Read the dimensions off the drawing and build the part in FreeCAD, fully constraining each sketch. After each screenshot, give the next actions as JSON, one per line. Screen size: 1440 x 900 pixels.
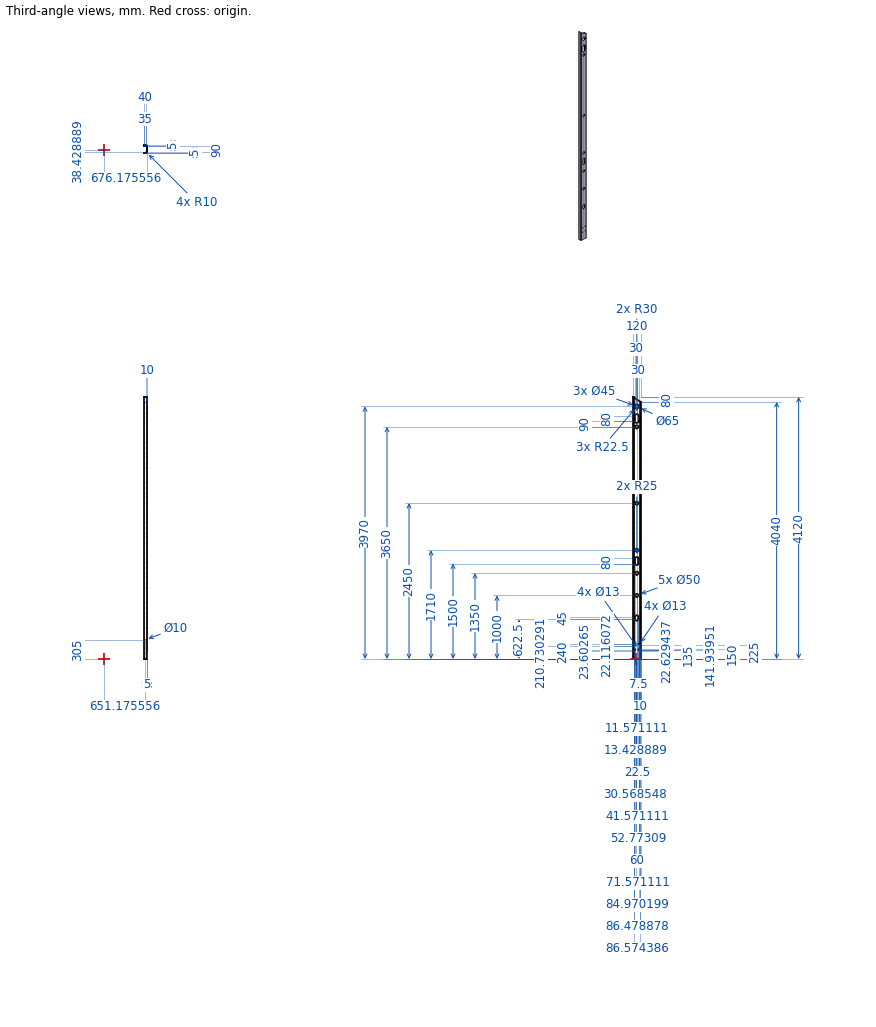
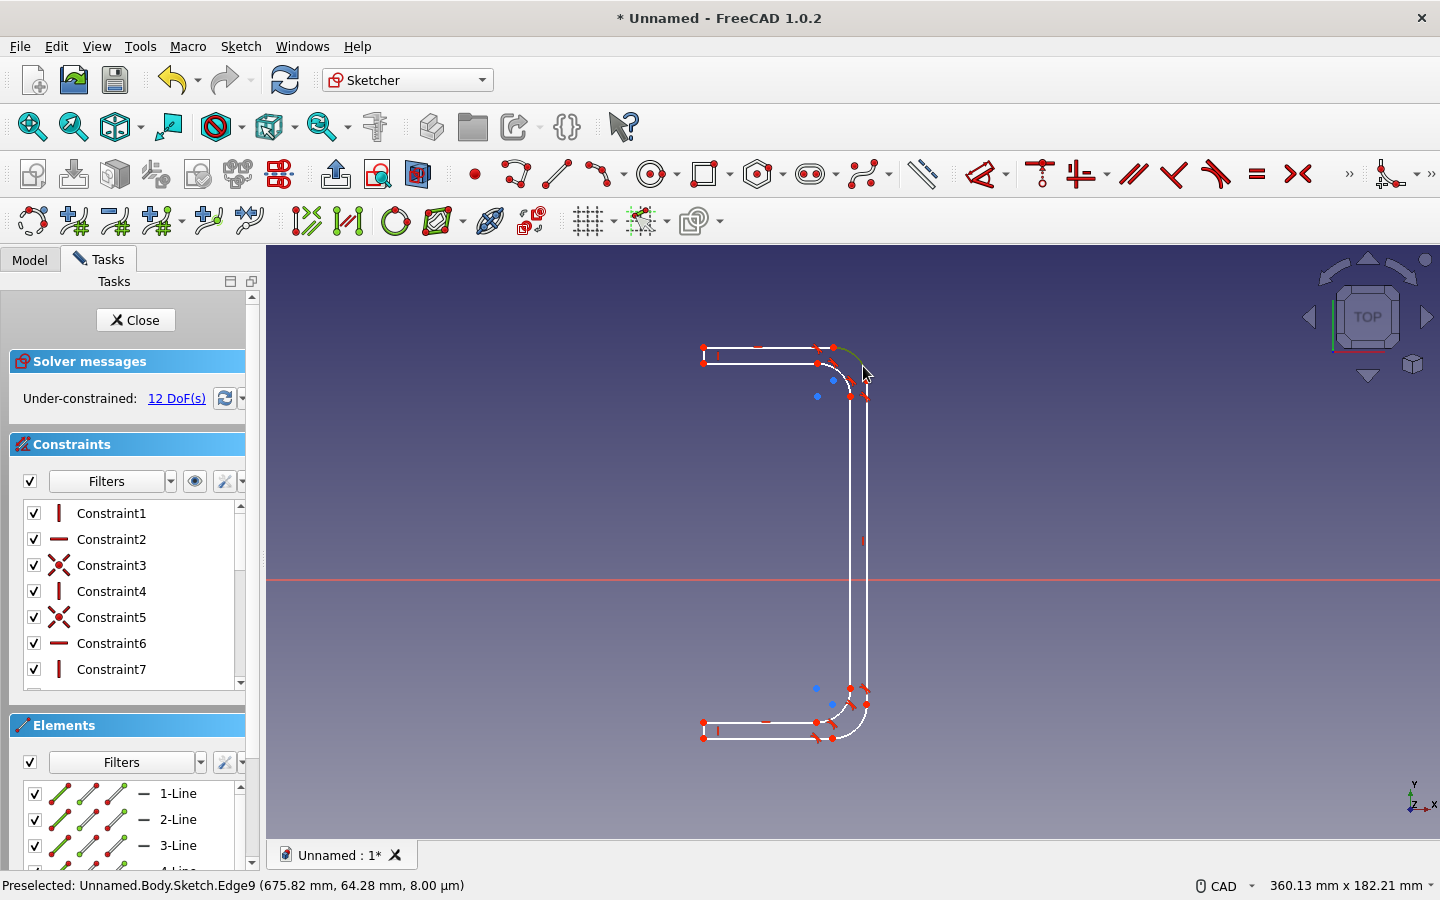
{"action": "left_click", "coordinate": [841, 373]}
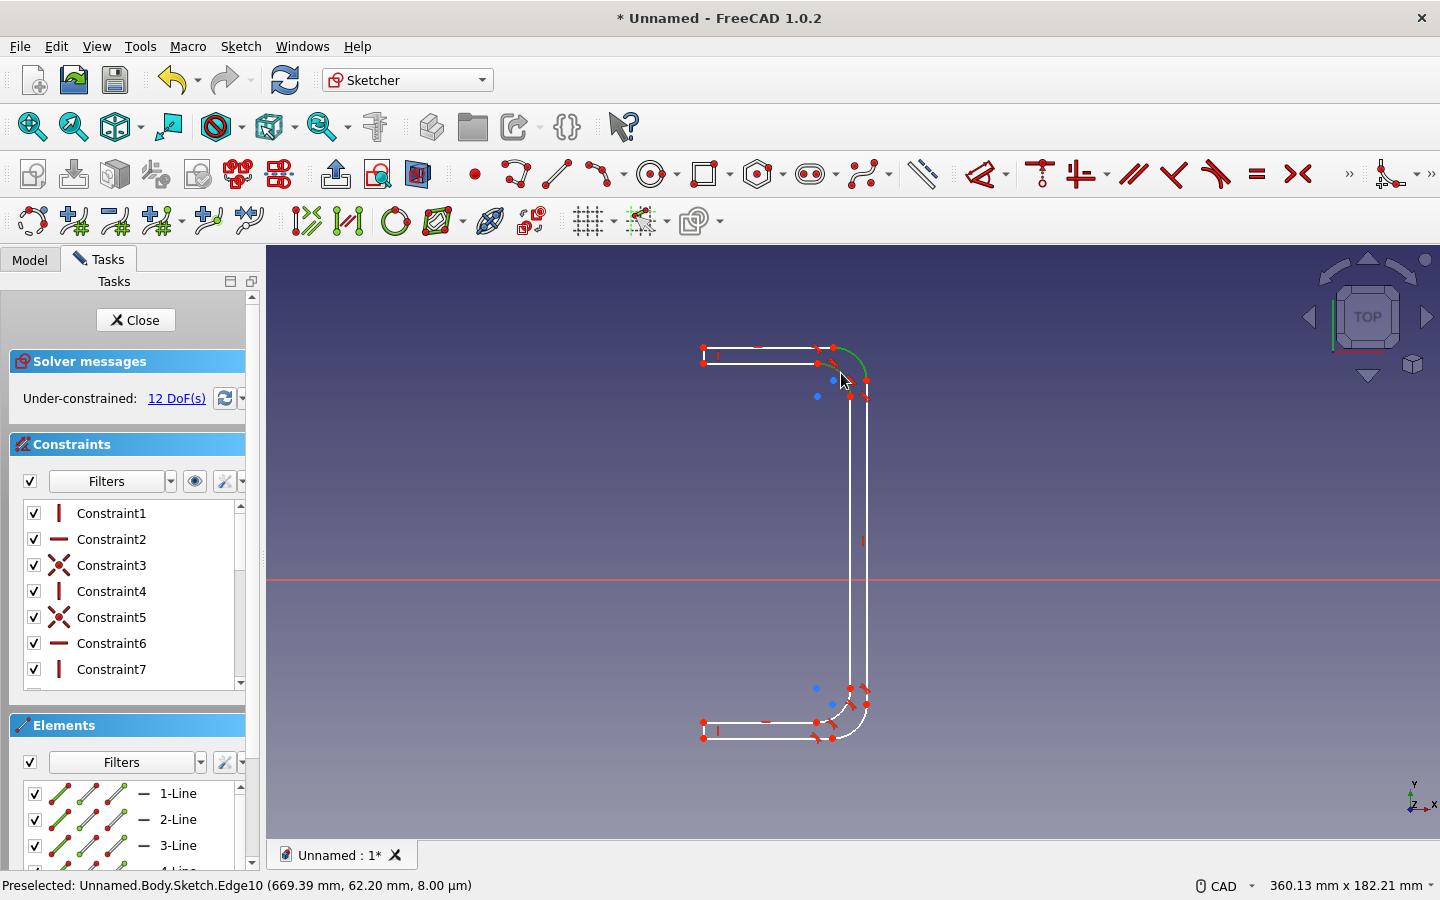
{"action": "left_click", "coordinate": [841, 713]}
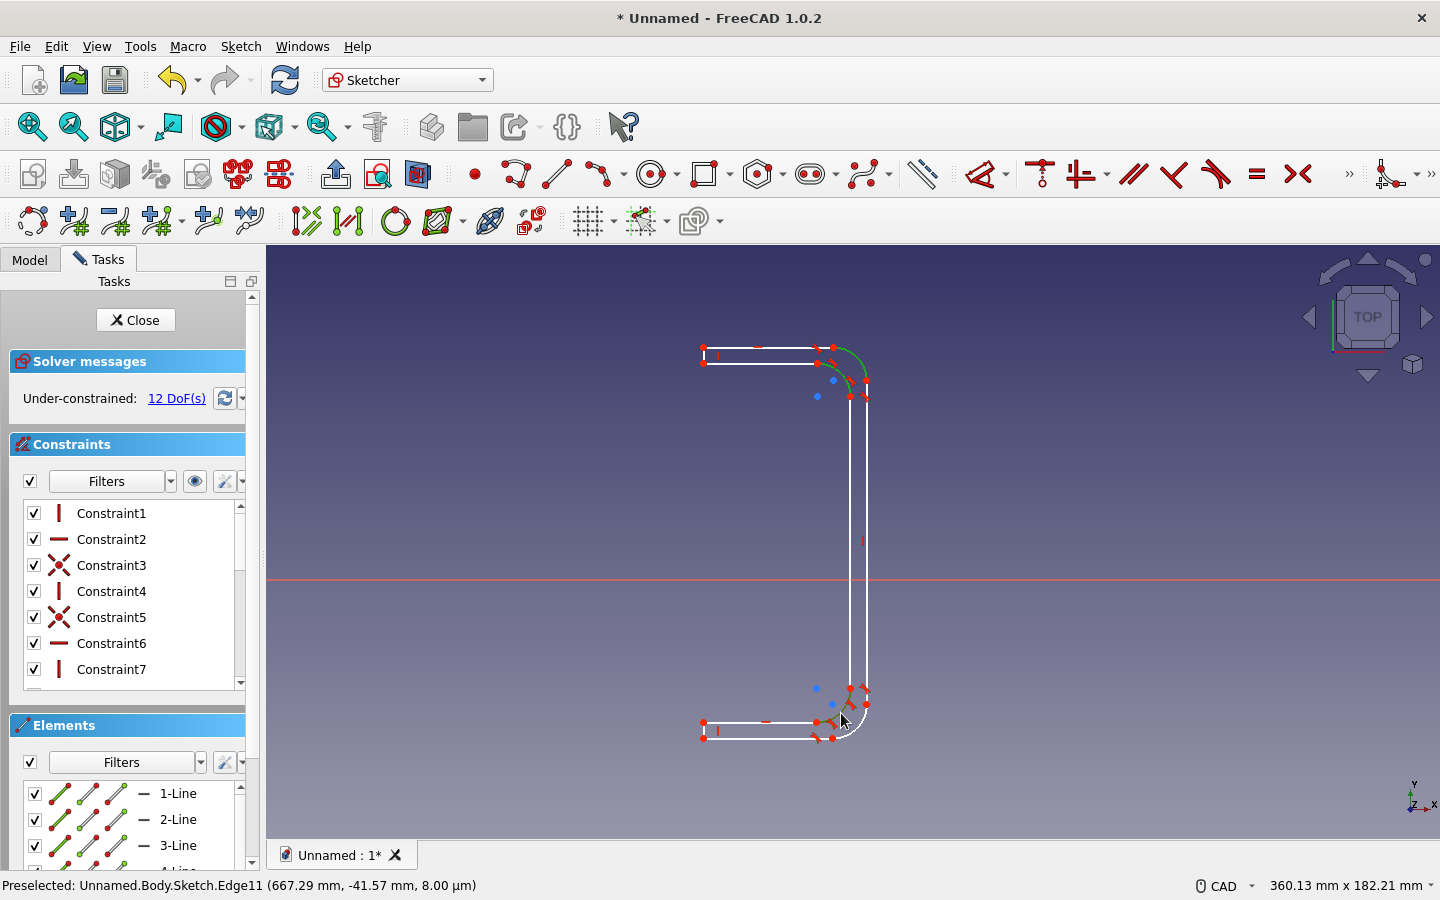
{"action": "left_click", "coordinate": [848, 735]}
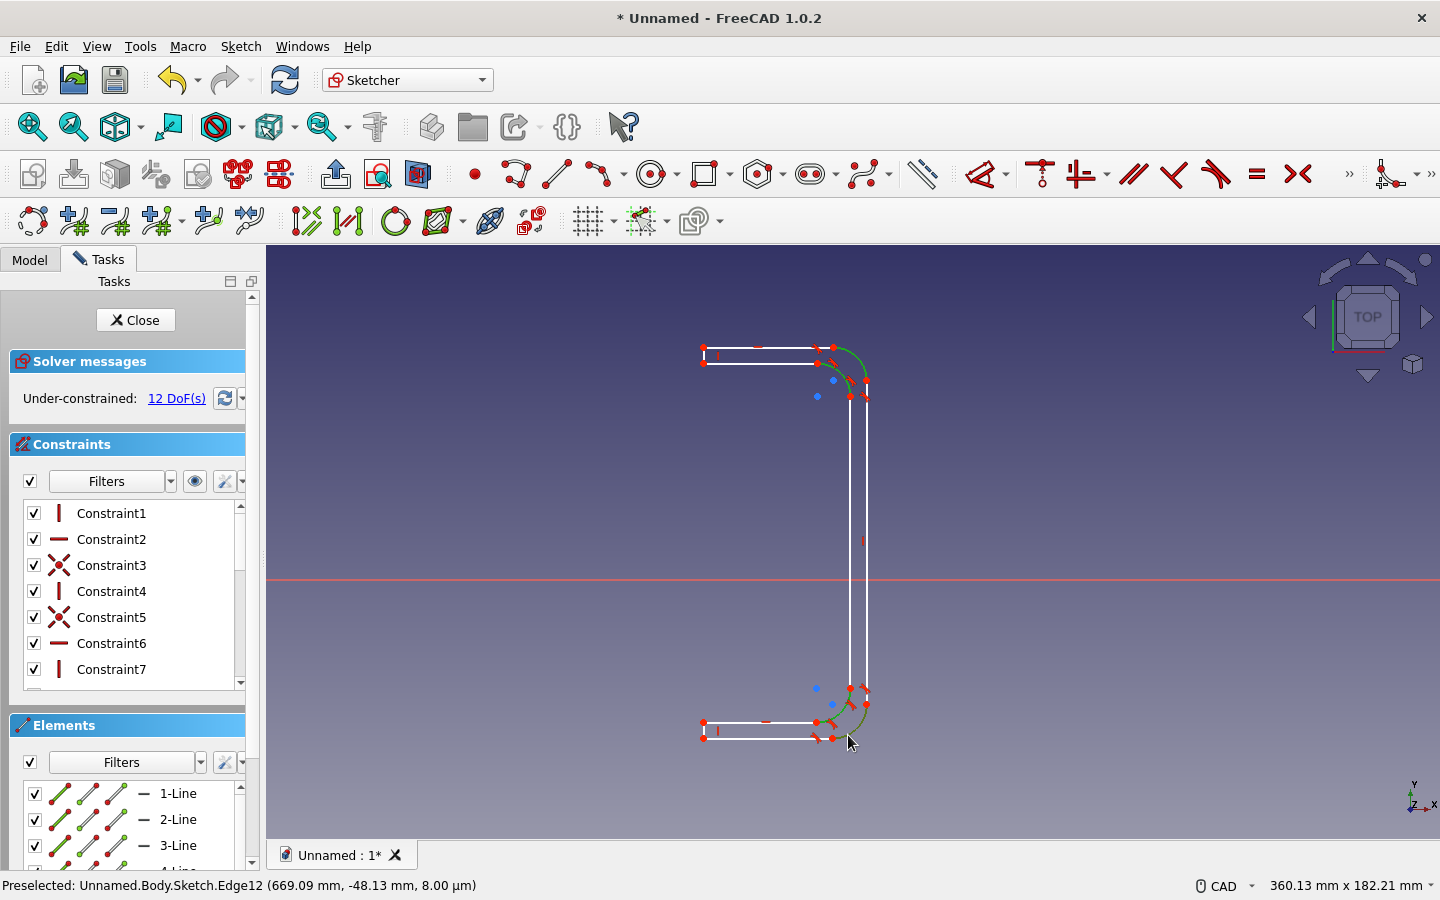
{"action": "left_click", "coordinate": [1257, 174]}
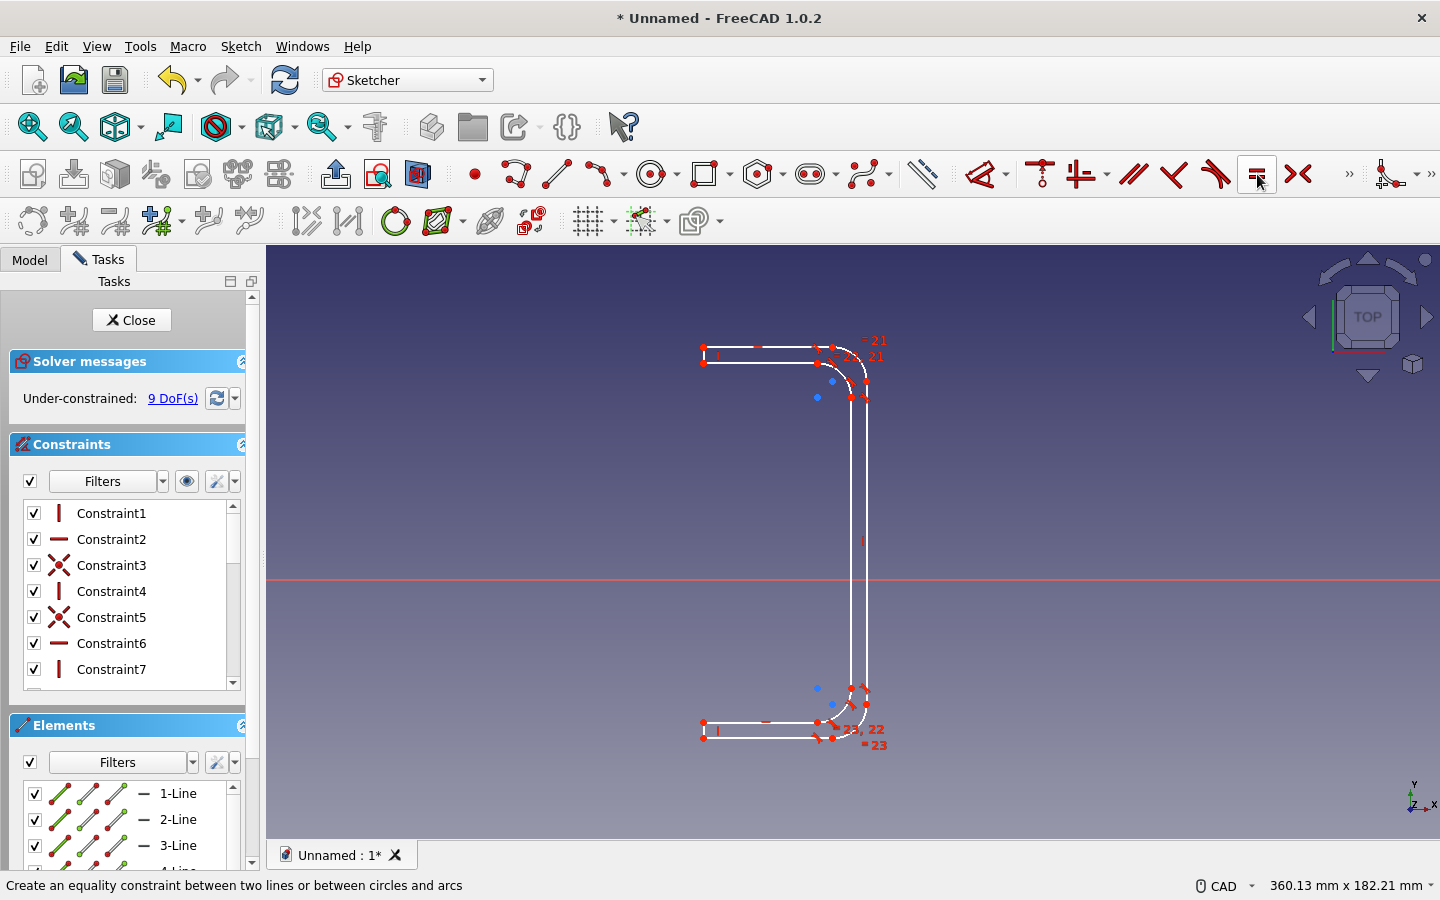
{"action": "key", "text": "d"}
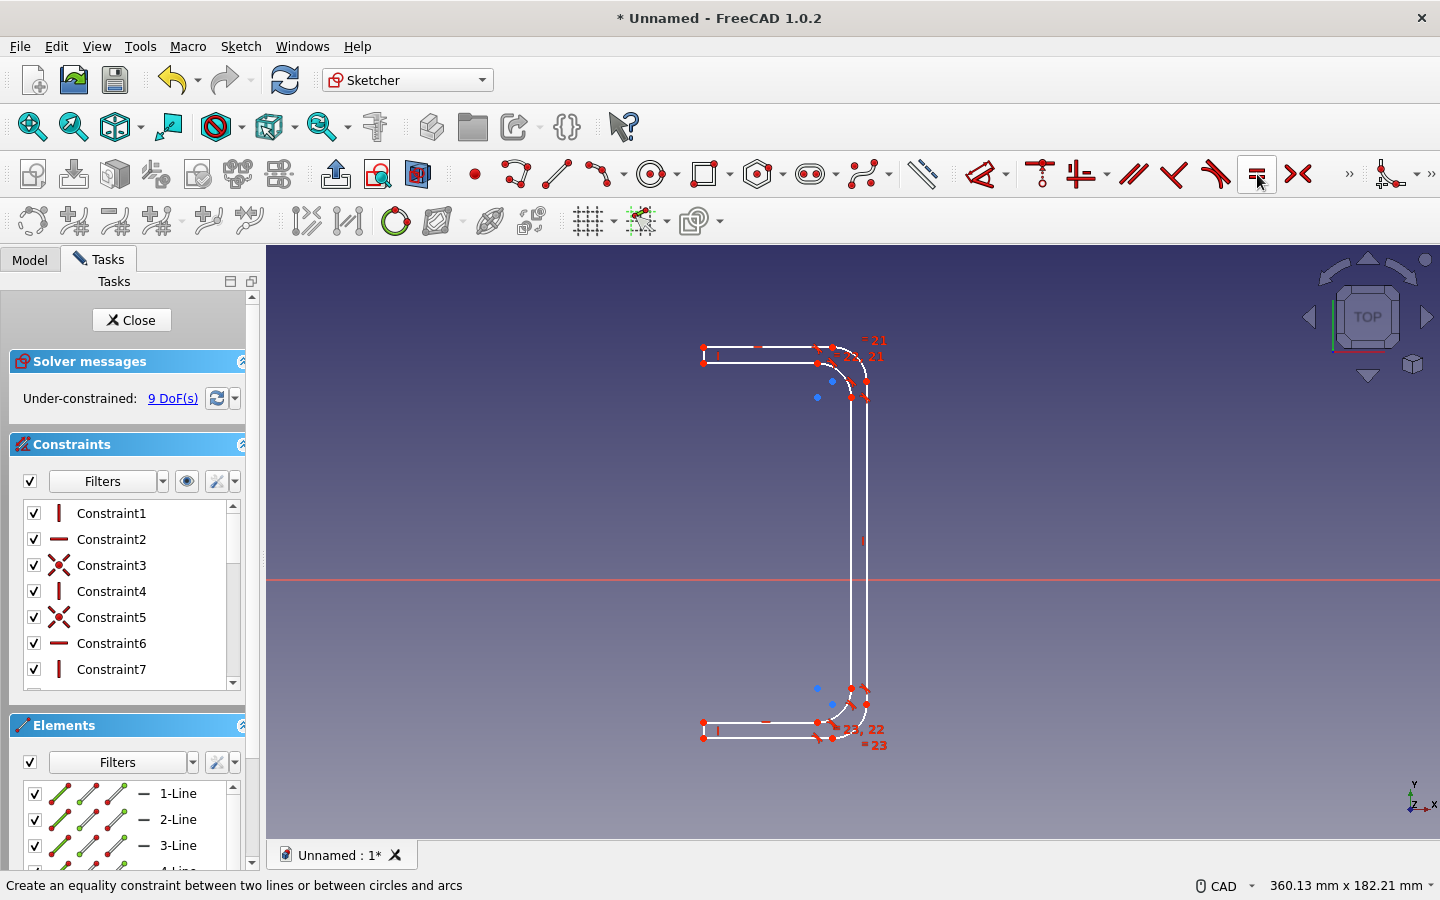
{"action": "left_click", "coordinate": [863, 366]}
{"action": "left_click", "coordinate": [892, 352]}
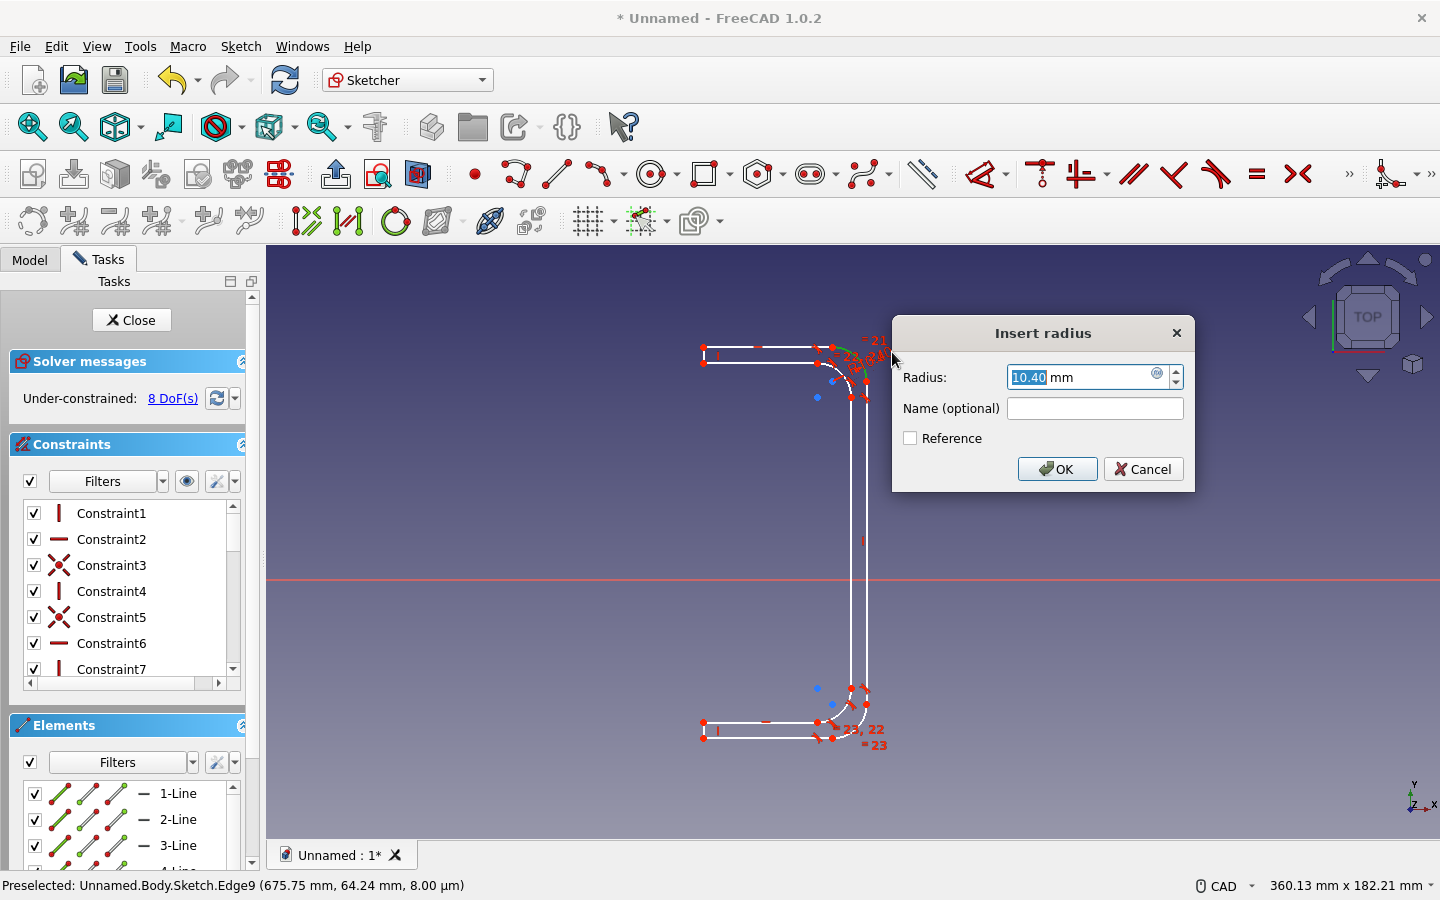
{"action": "type", "text": "10"}
{"action": "key", "text": "Return"}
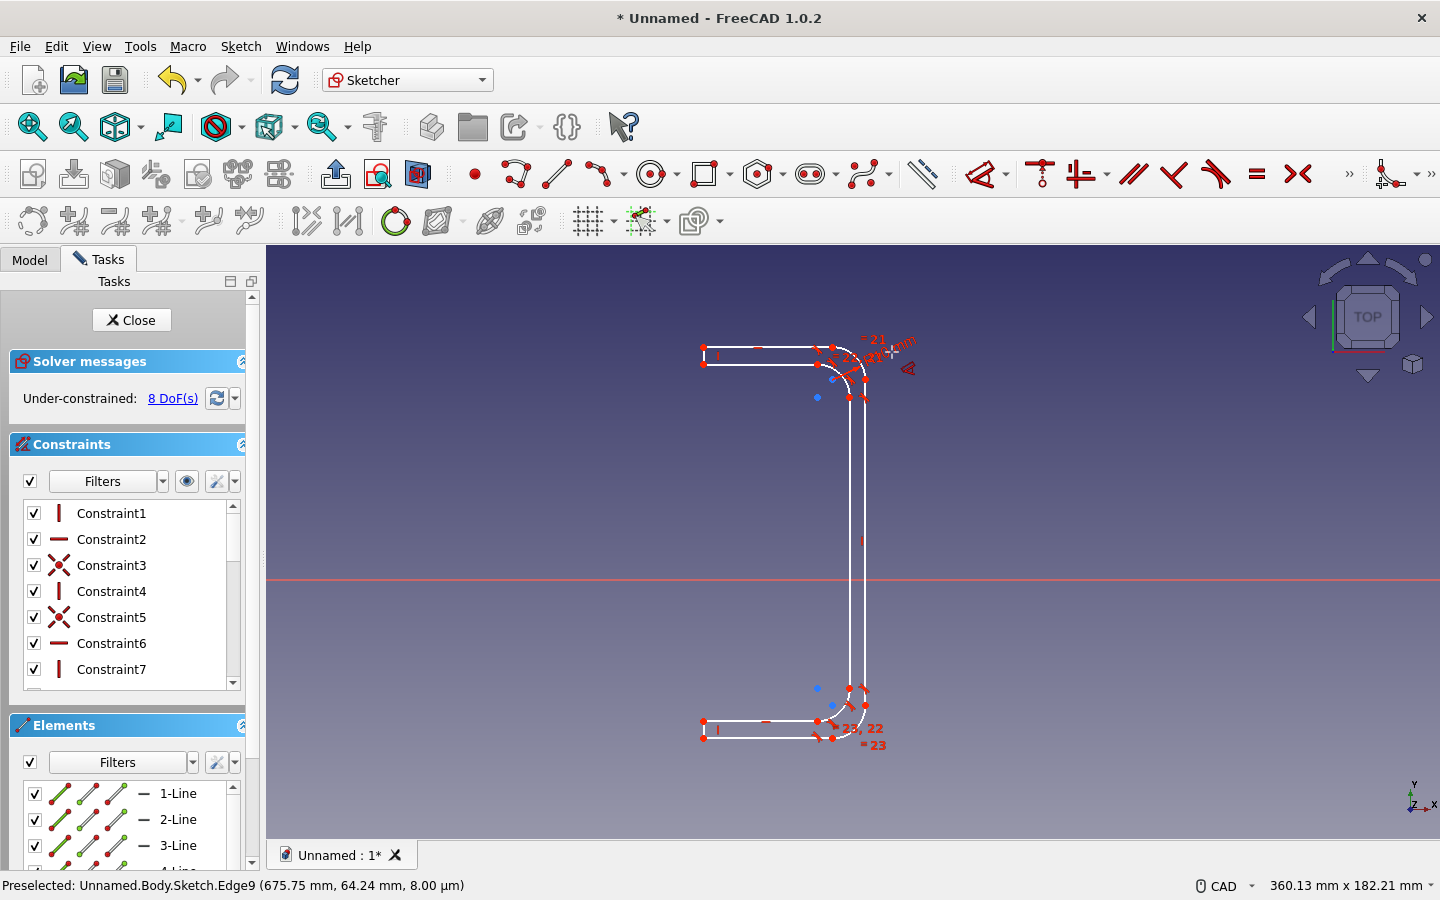
{"action": "scroll", "coordinate": [704, 356], "scroll_direction": "up", "scroll_amount": 5}